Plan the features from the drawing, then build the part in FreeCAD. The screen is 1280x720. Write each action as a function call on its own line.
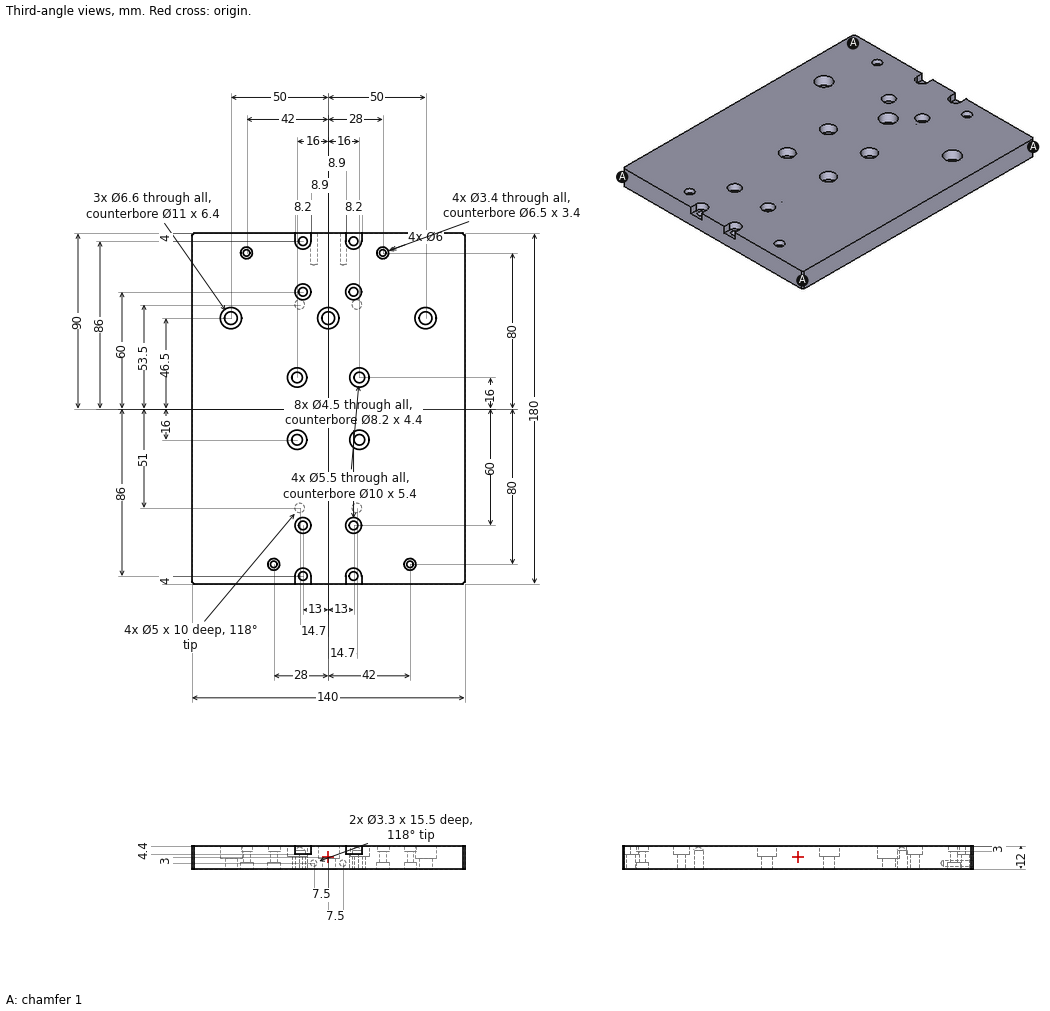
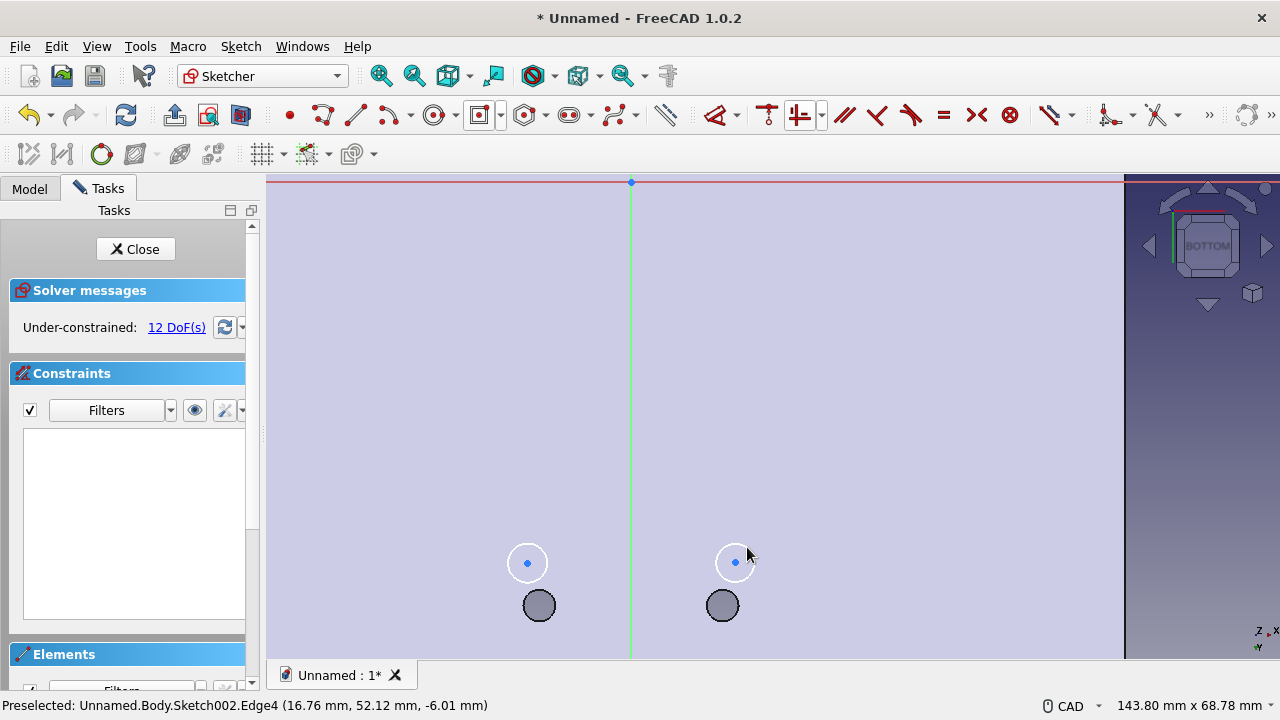
scroll(747, 548, down, 5)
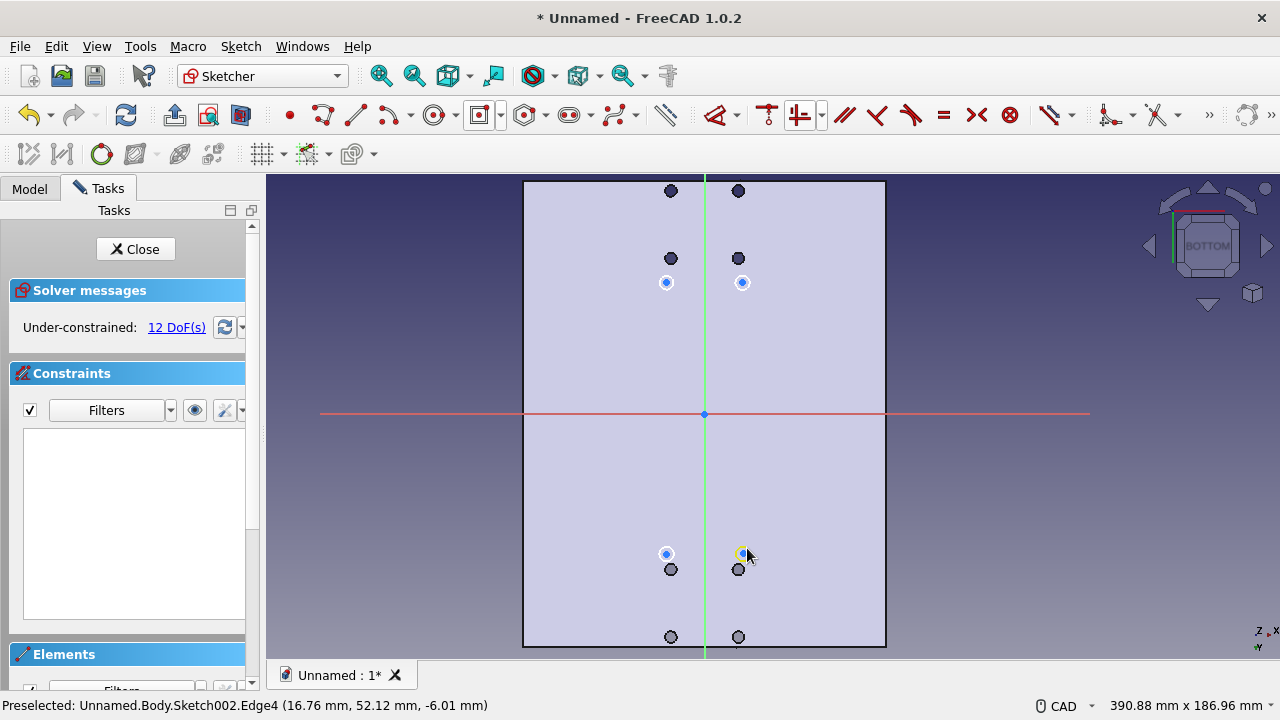
scroll(671, 278, up, 4)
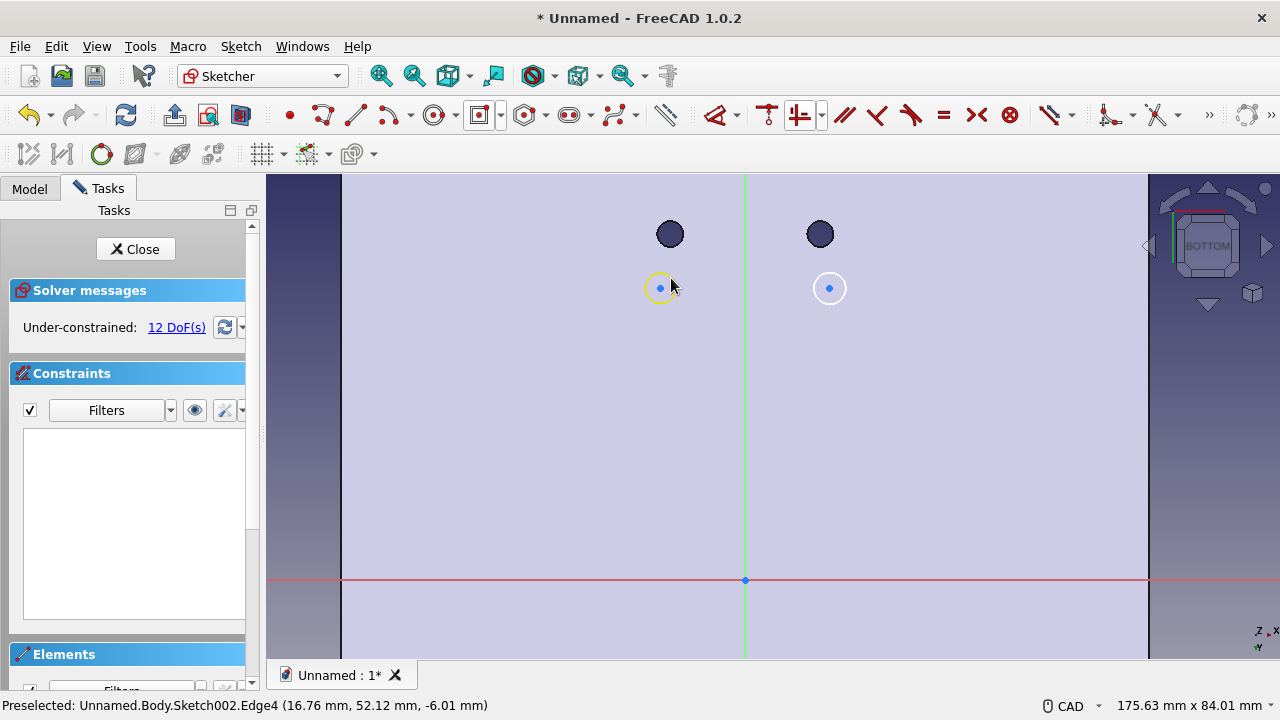
click(671, 277)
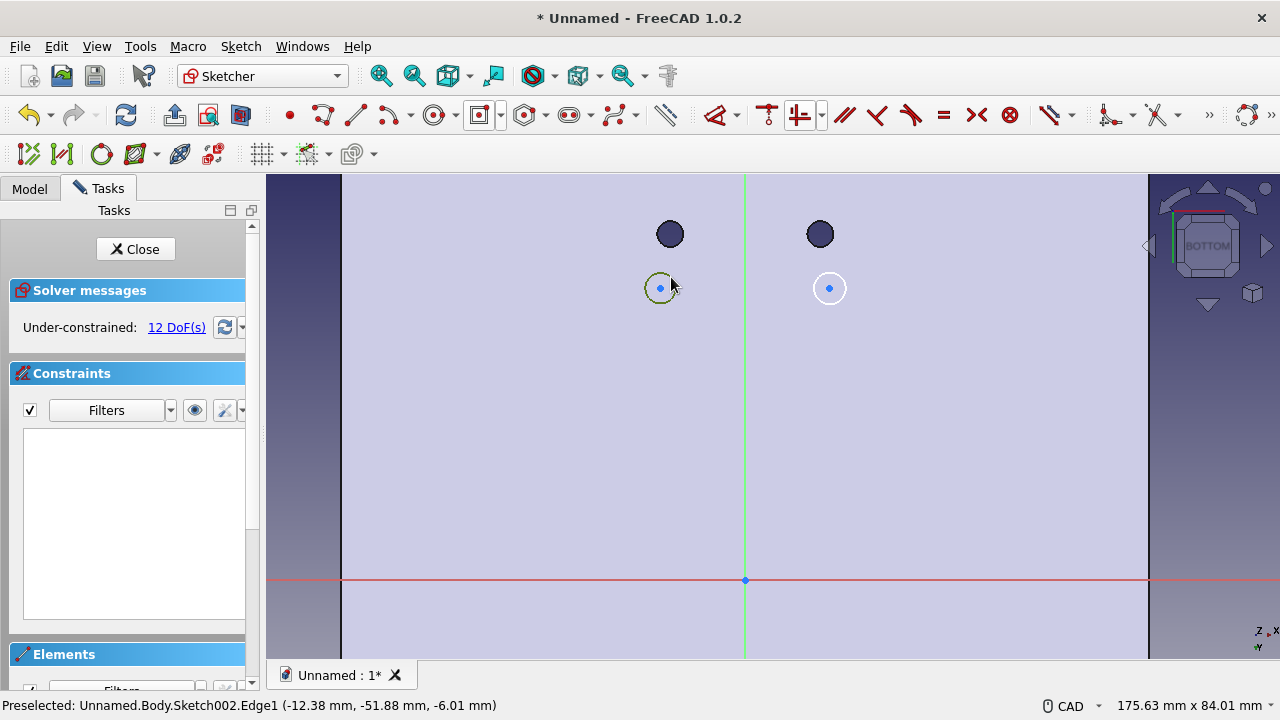
click(841, 277)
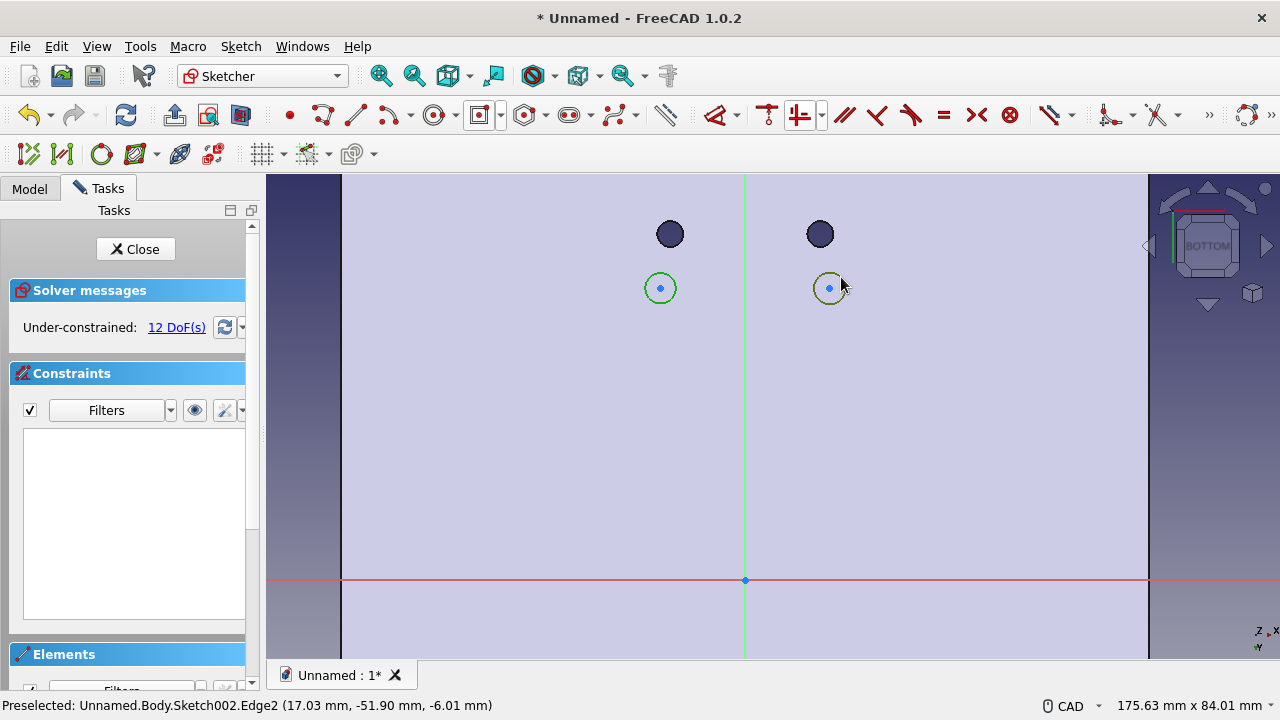
scroll(671, 277, down, 4)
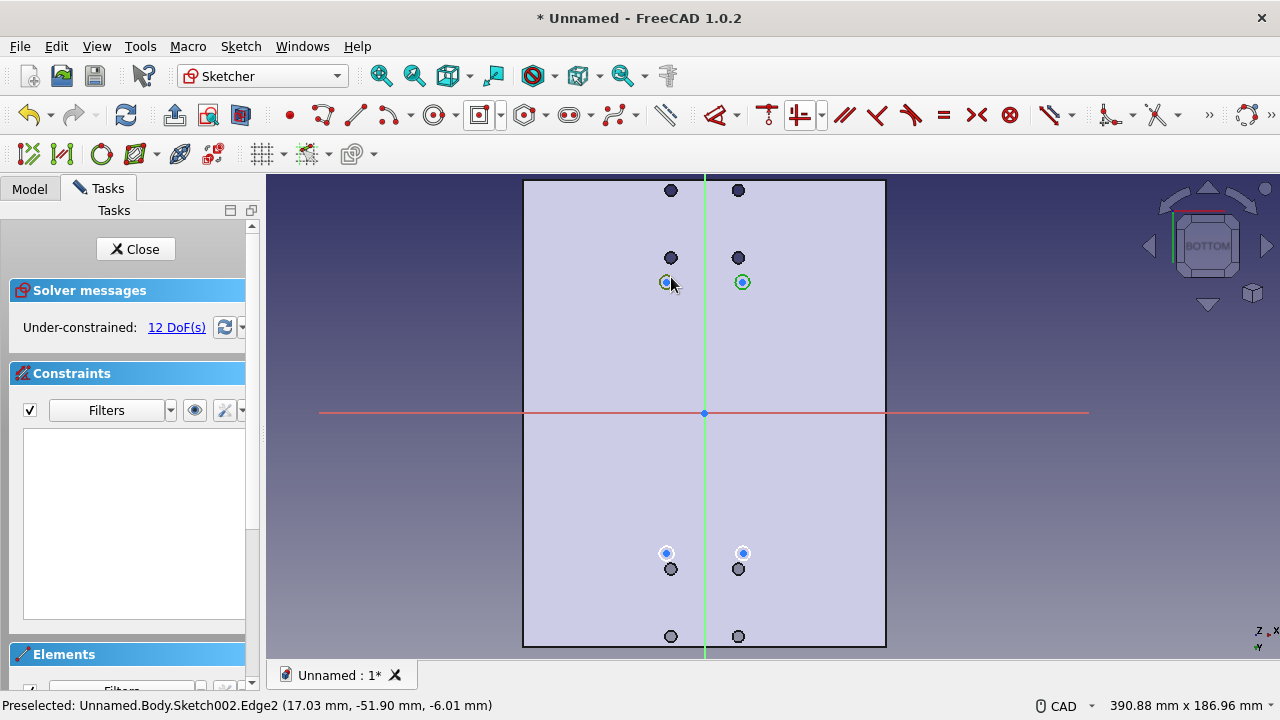
scroll(672, 548, up, 4)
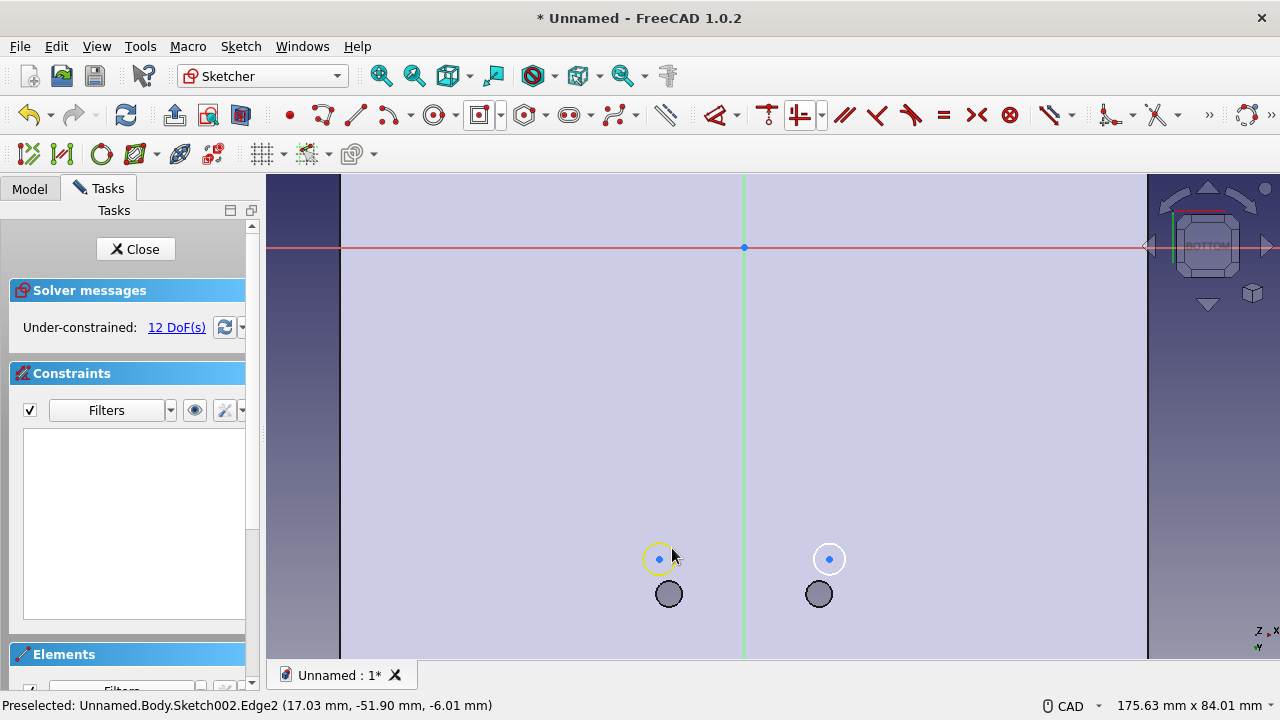
click(671, 548)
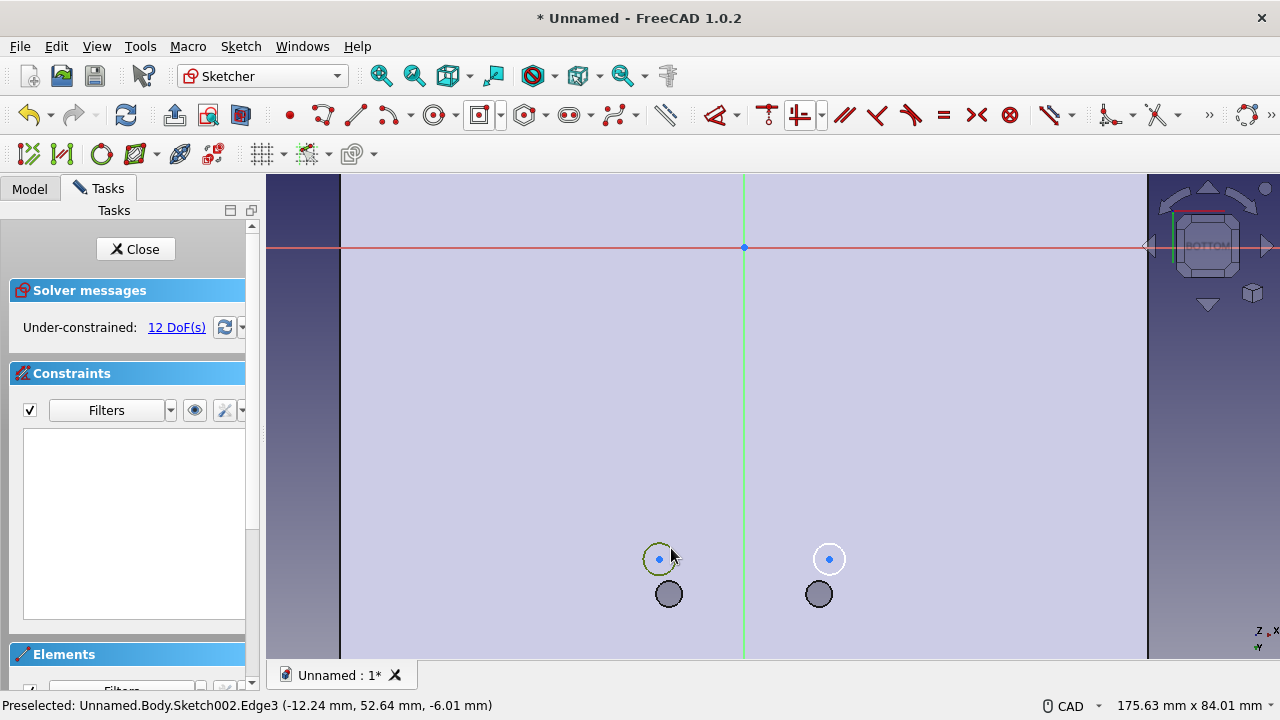
click(840, 548)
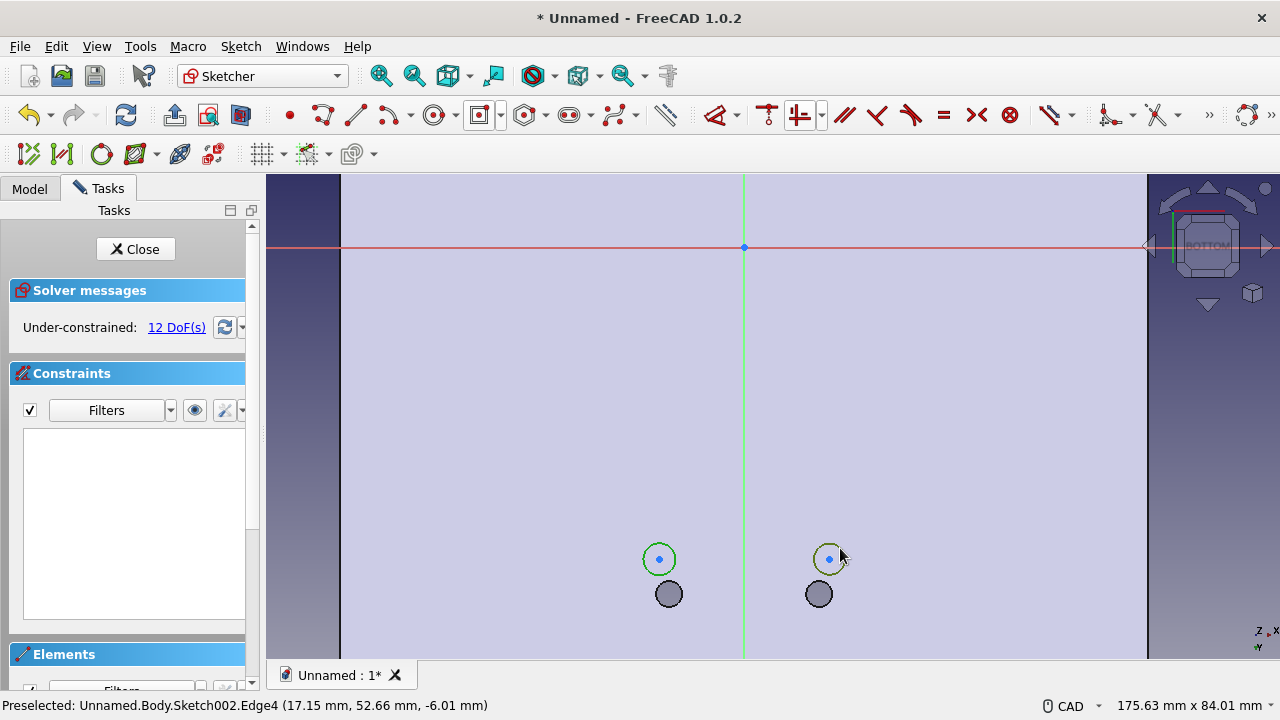
click(944, 116)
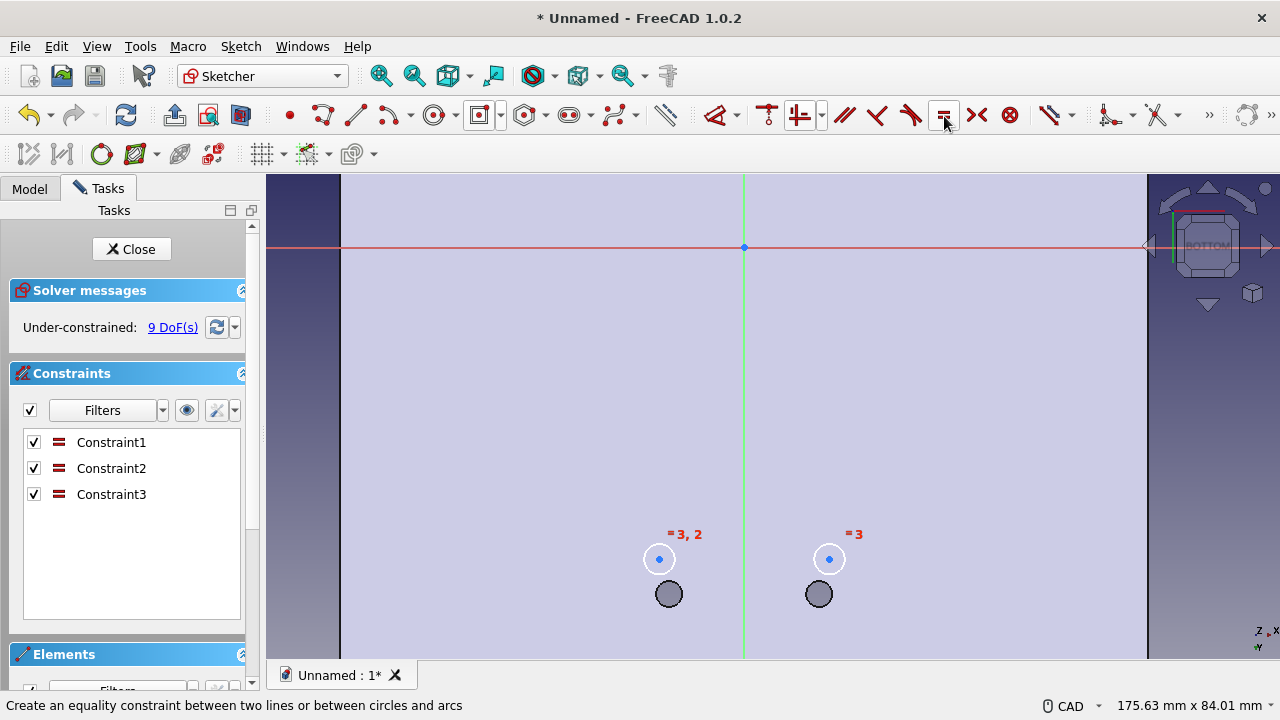
click(714, 116)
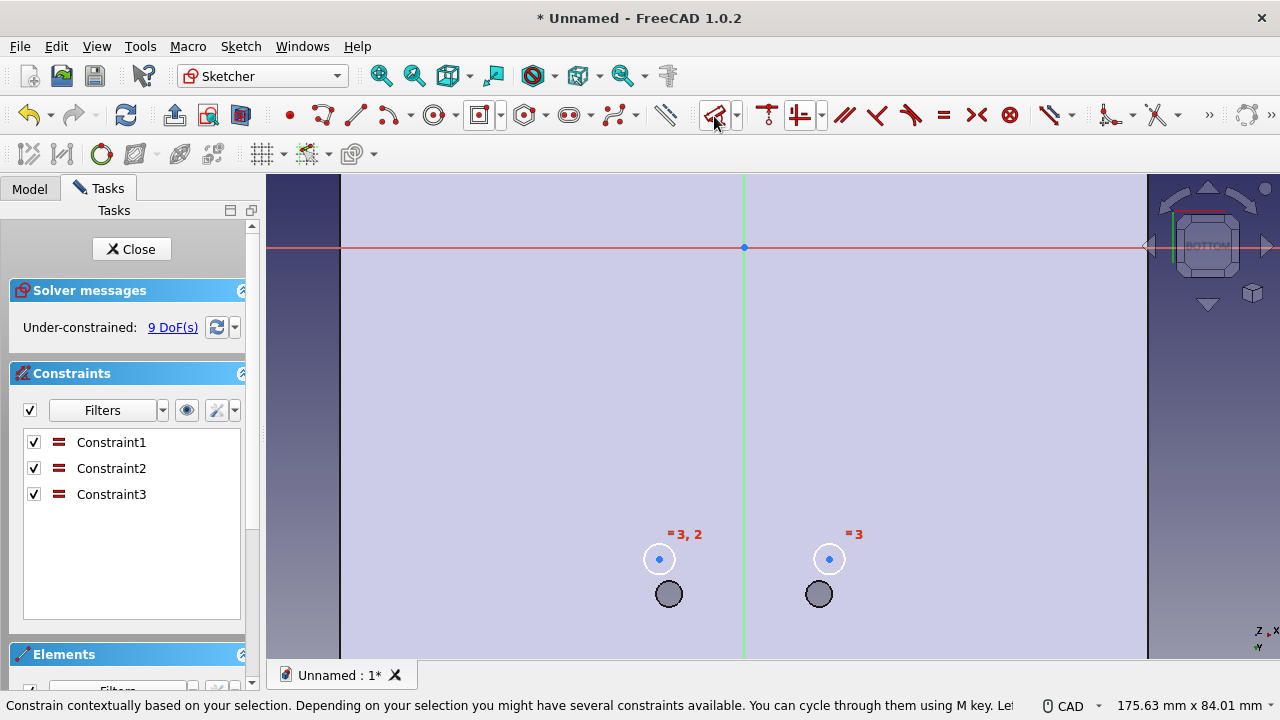
scroll(672, 548, down, 4)